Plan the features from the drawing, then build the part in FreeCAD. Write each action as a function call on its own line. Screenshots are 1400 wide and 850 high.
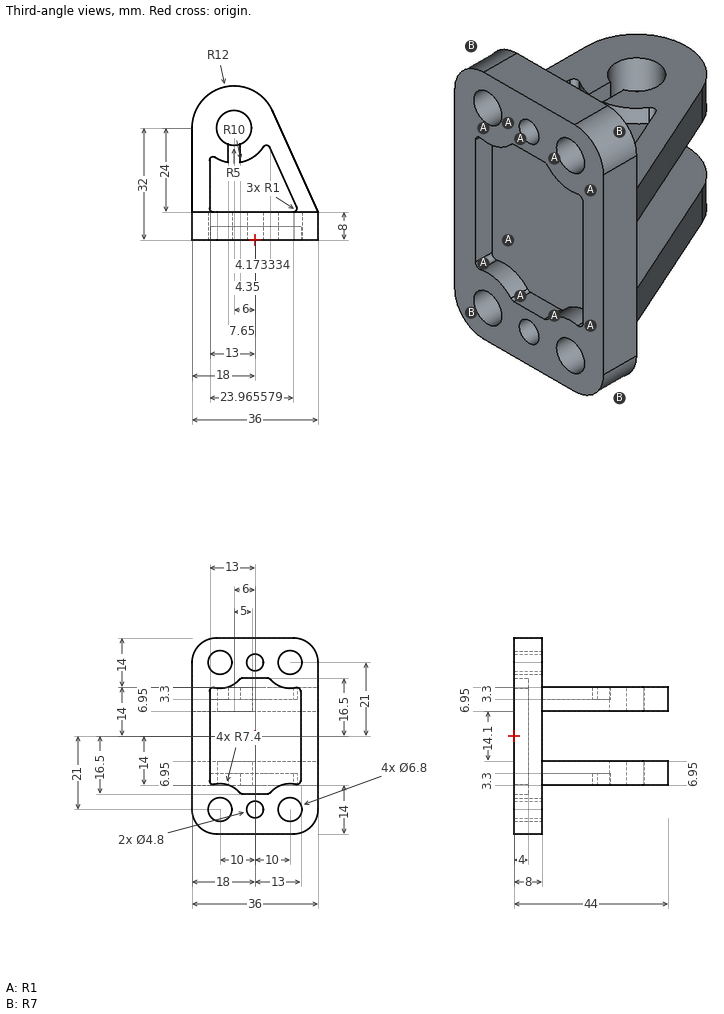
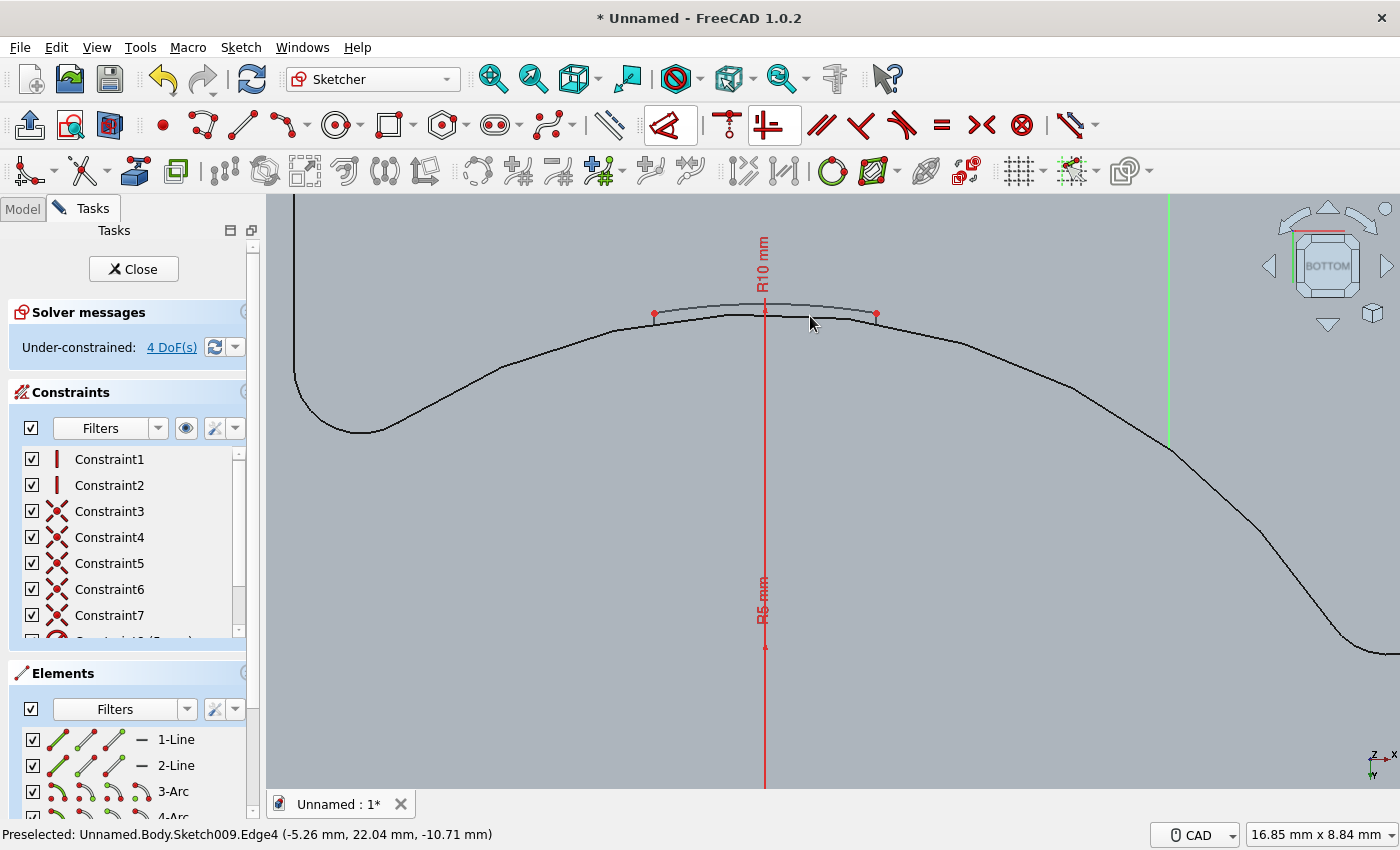
scroll(764, 304, down, 3)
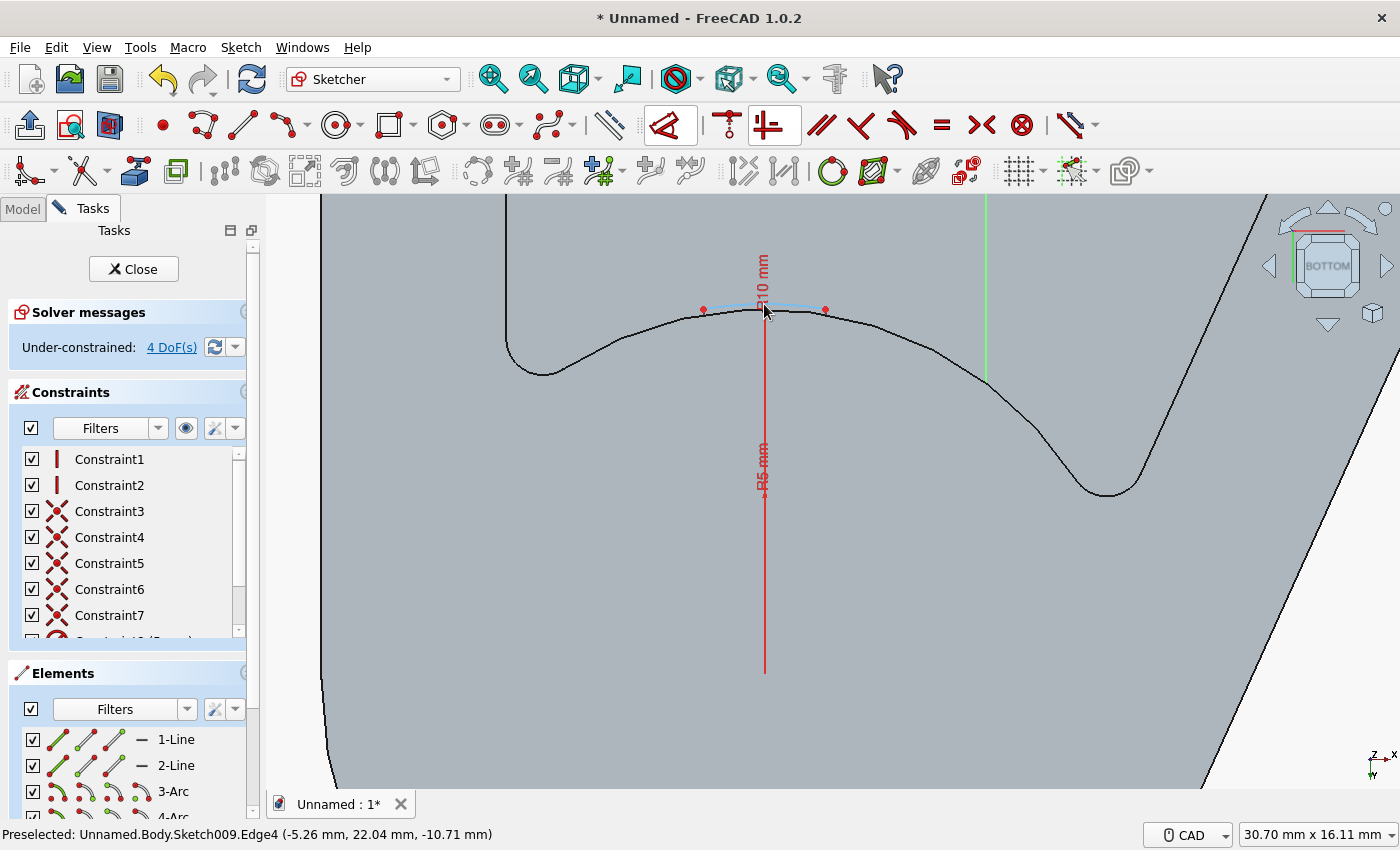
click(765, 673)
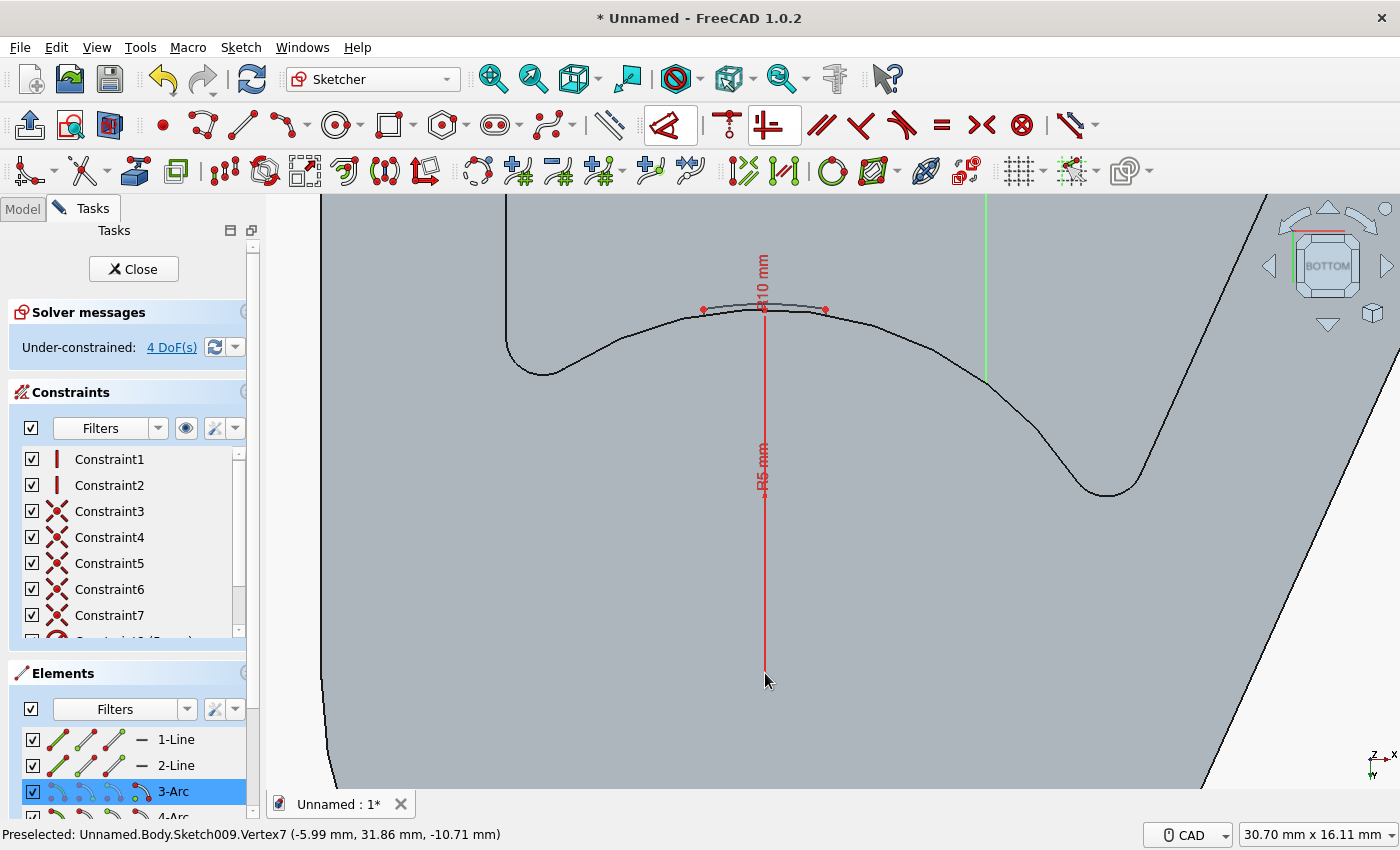
key(l)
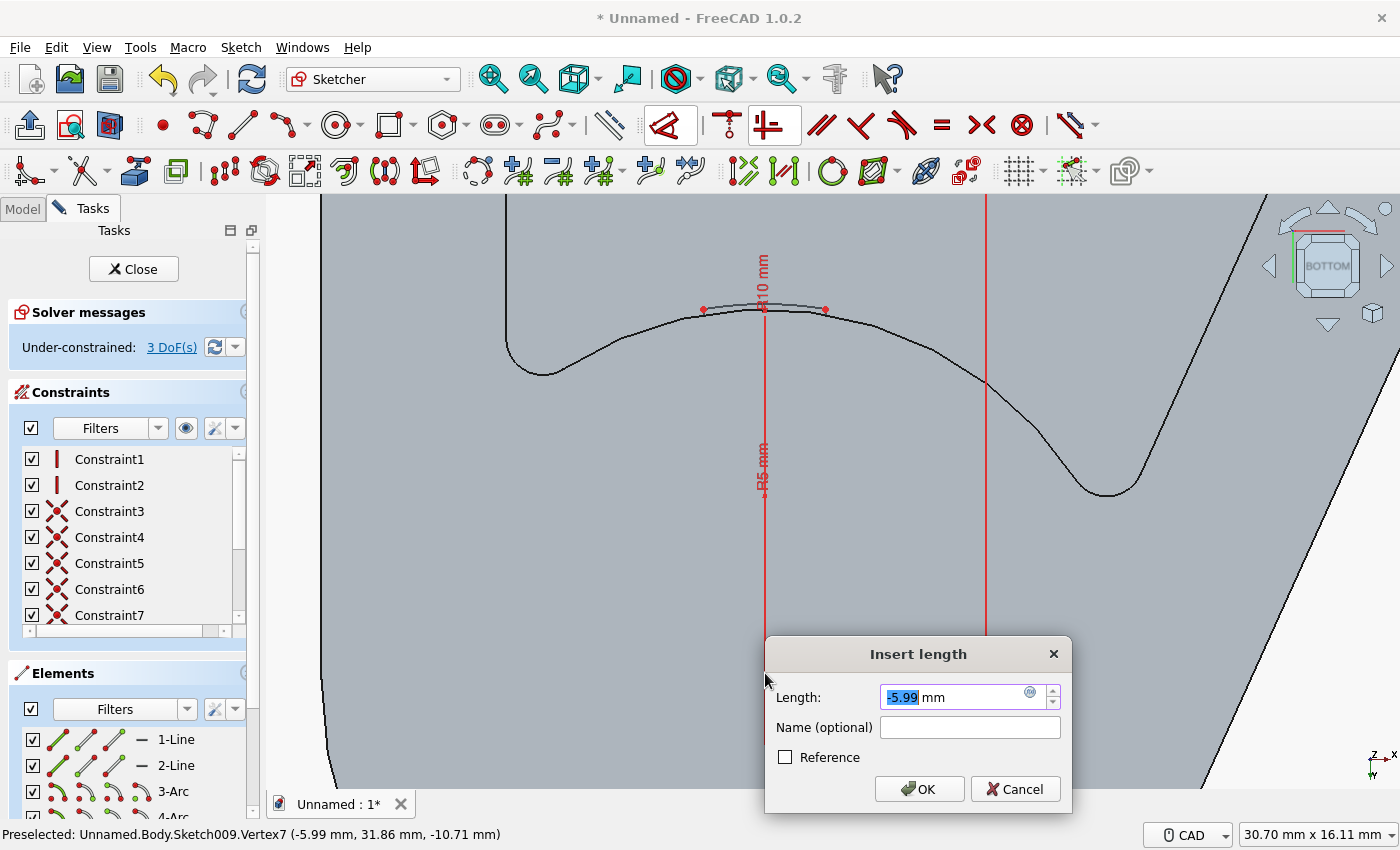
text(-6)
key(Return)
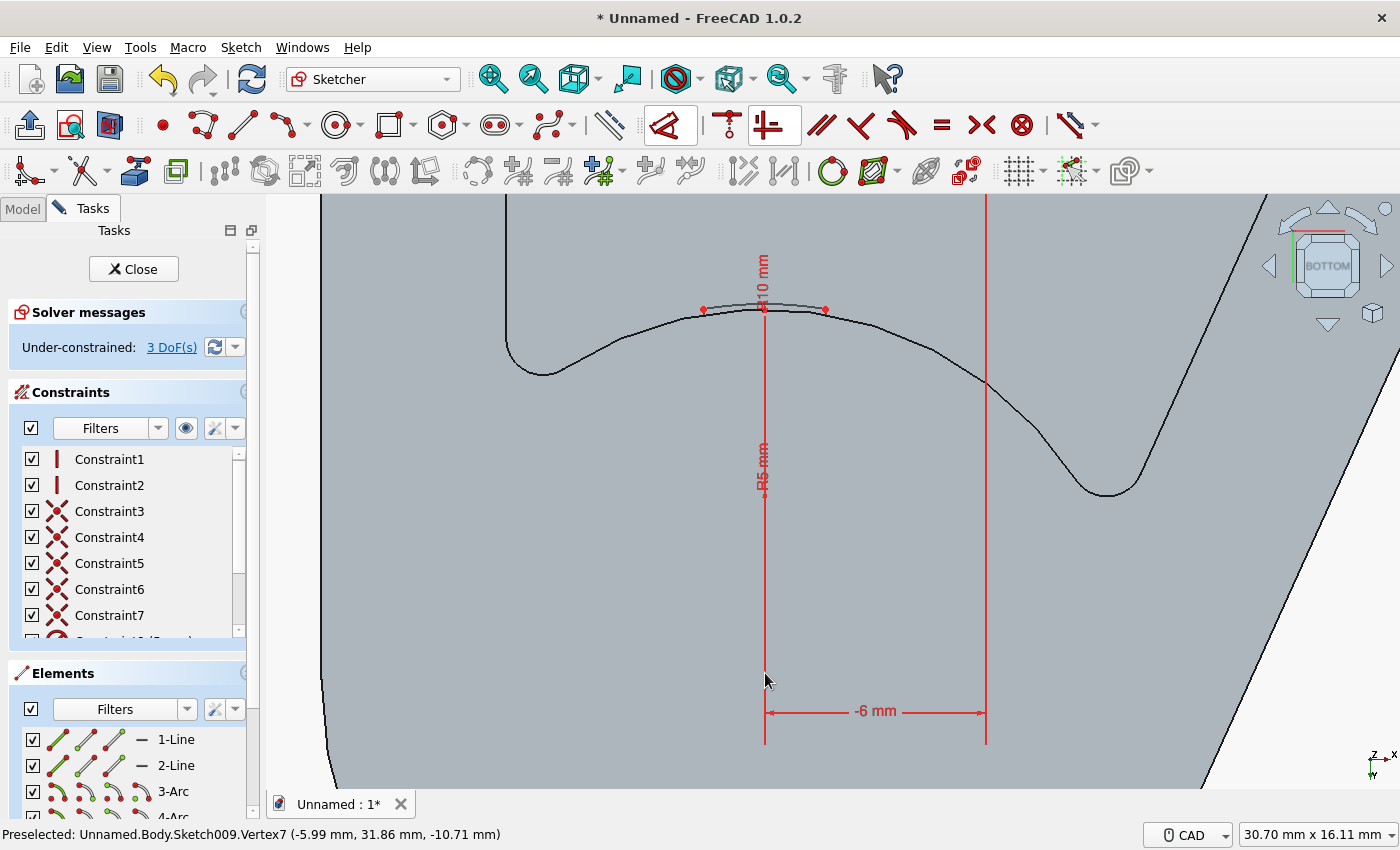
click(765, 673)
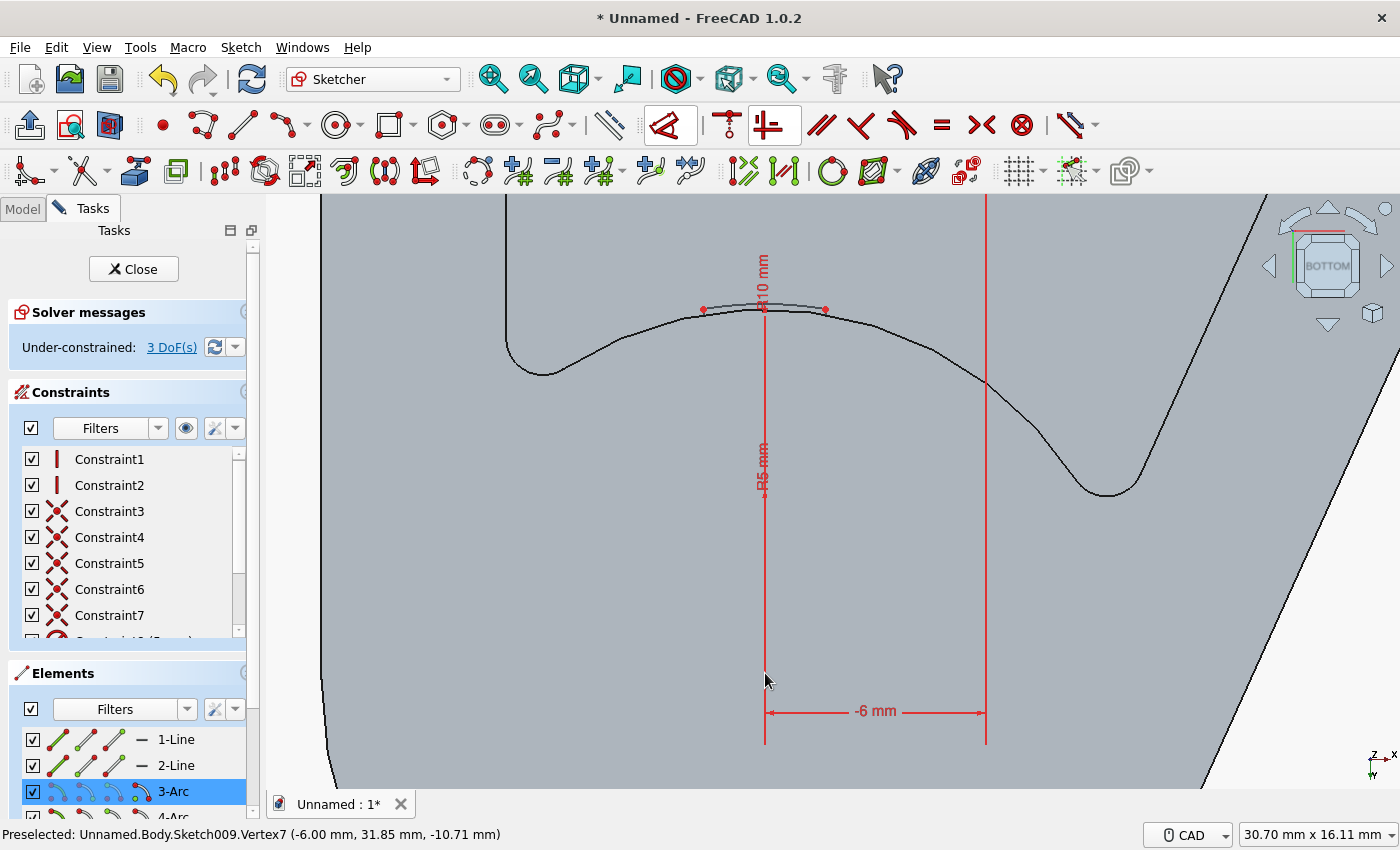
key(i)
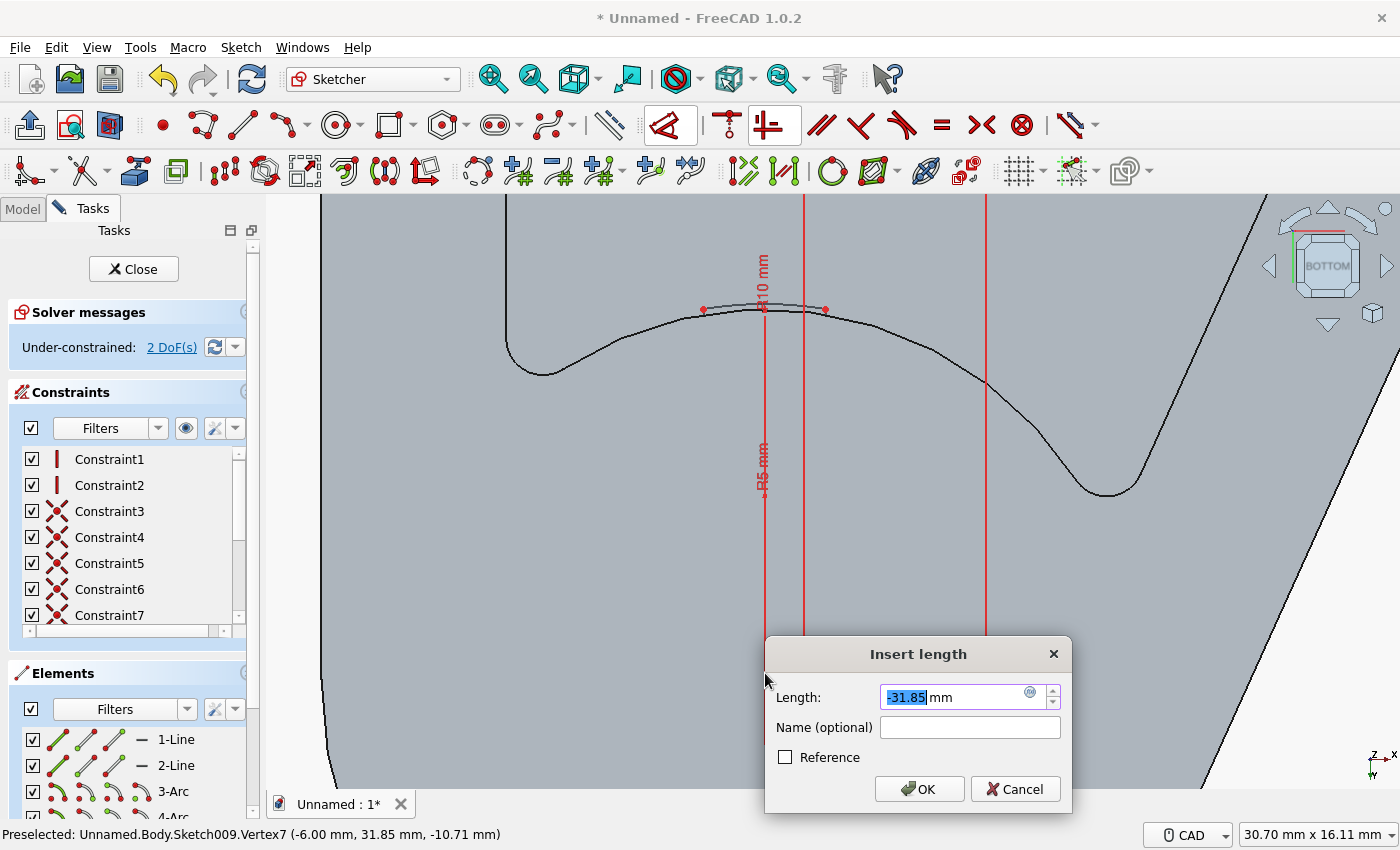
text(-32)
key(Return)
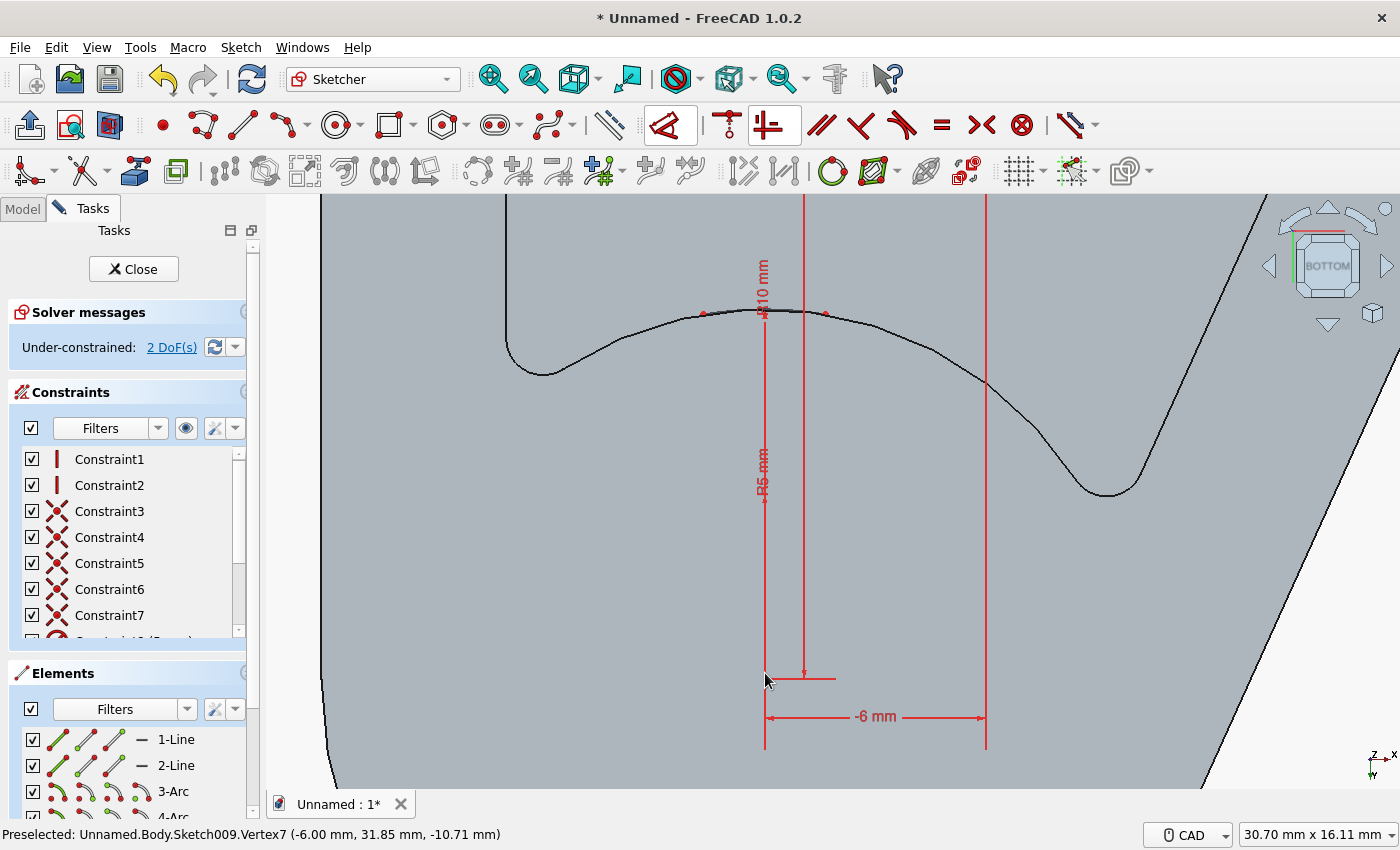
click(704, 314)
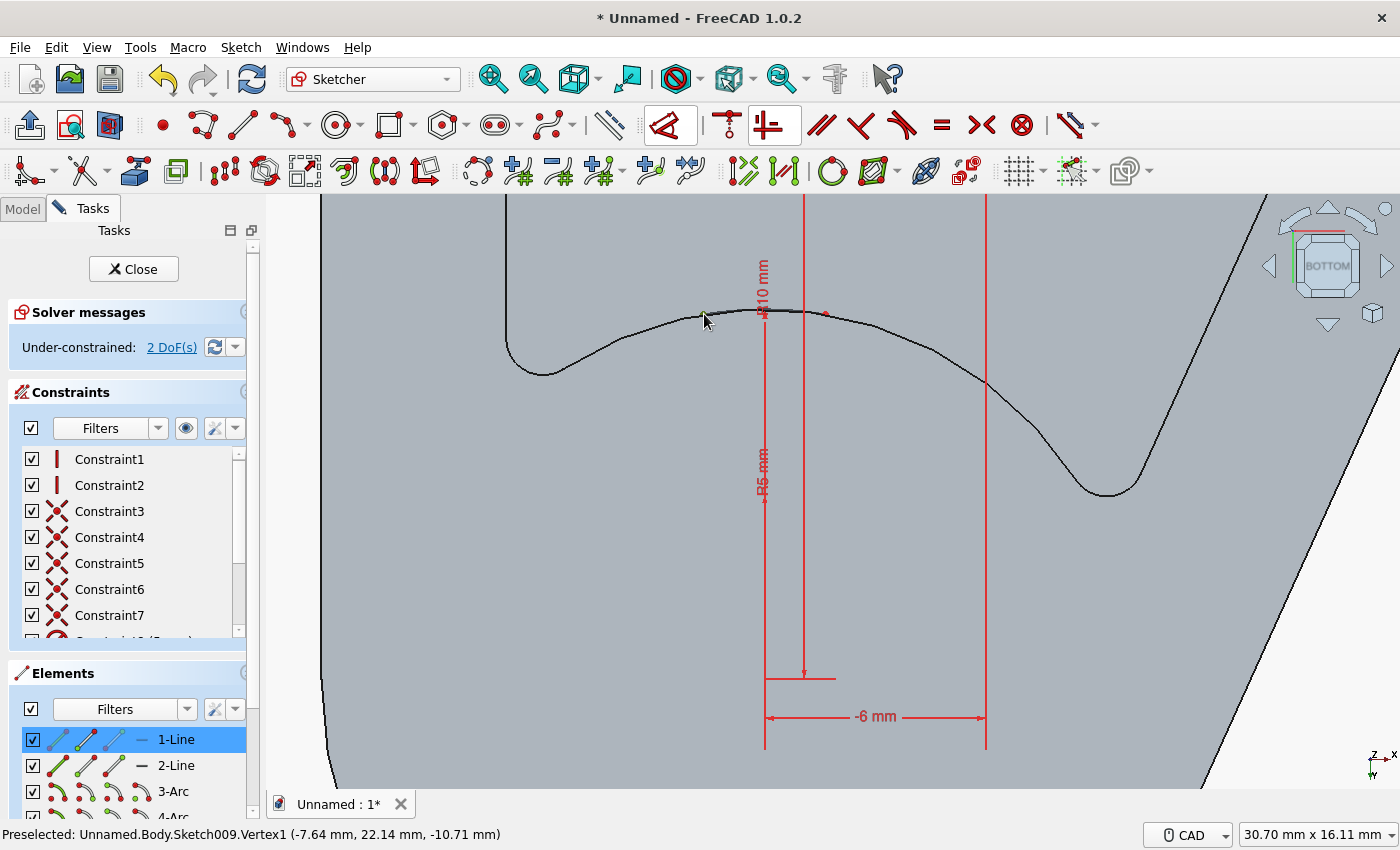
key(l)